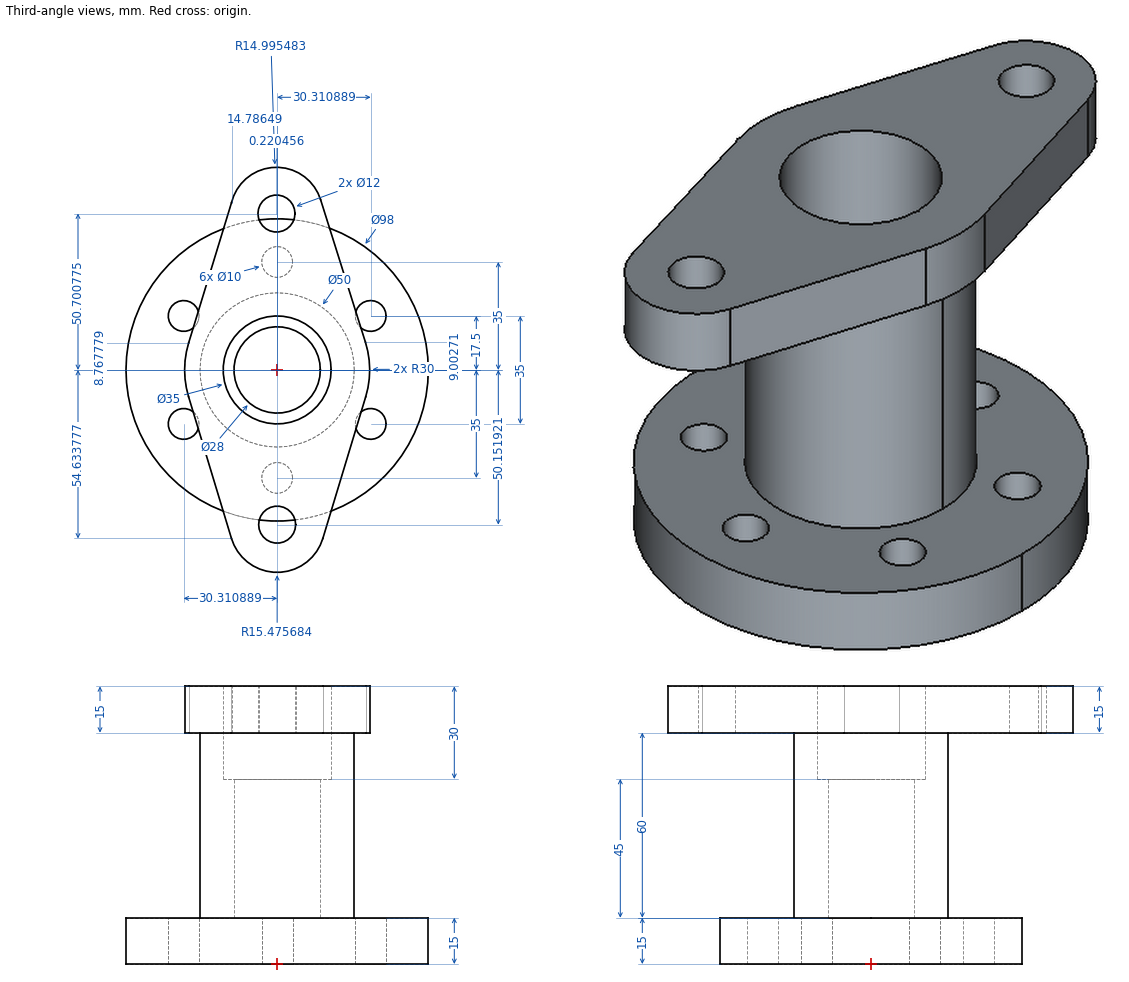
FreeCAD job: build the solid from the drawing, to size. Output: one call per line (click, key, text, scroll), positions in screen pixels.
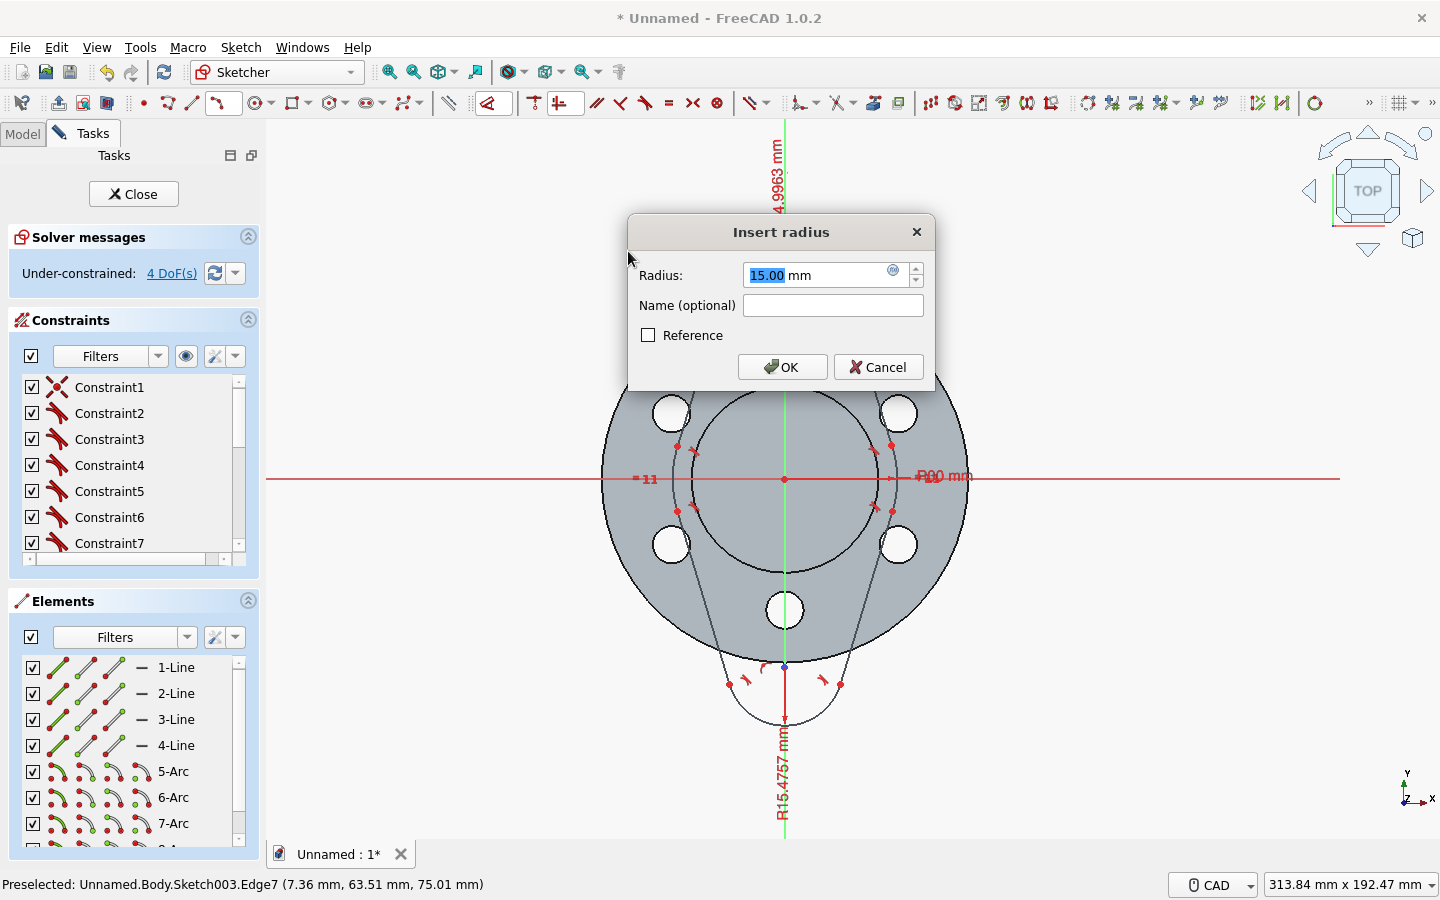
text(14.995483)
key(Return)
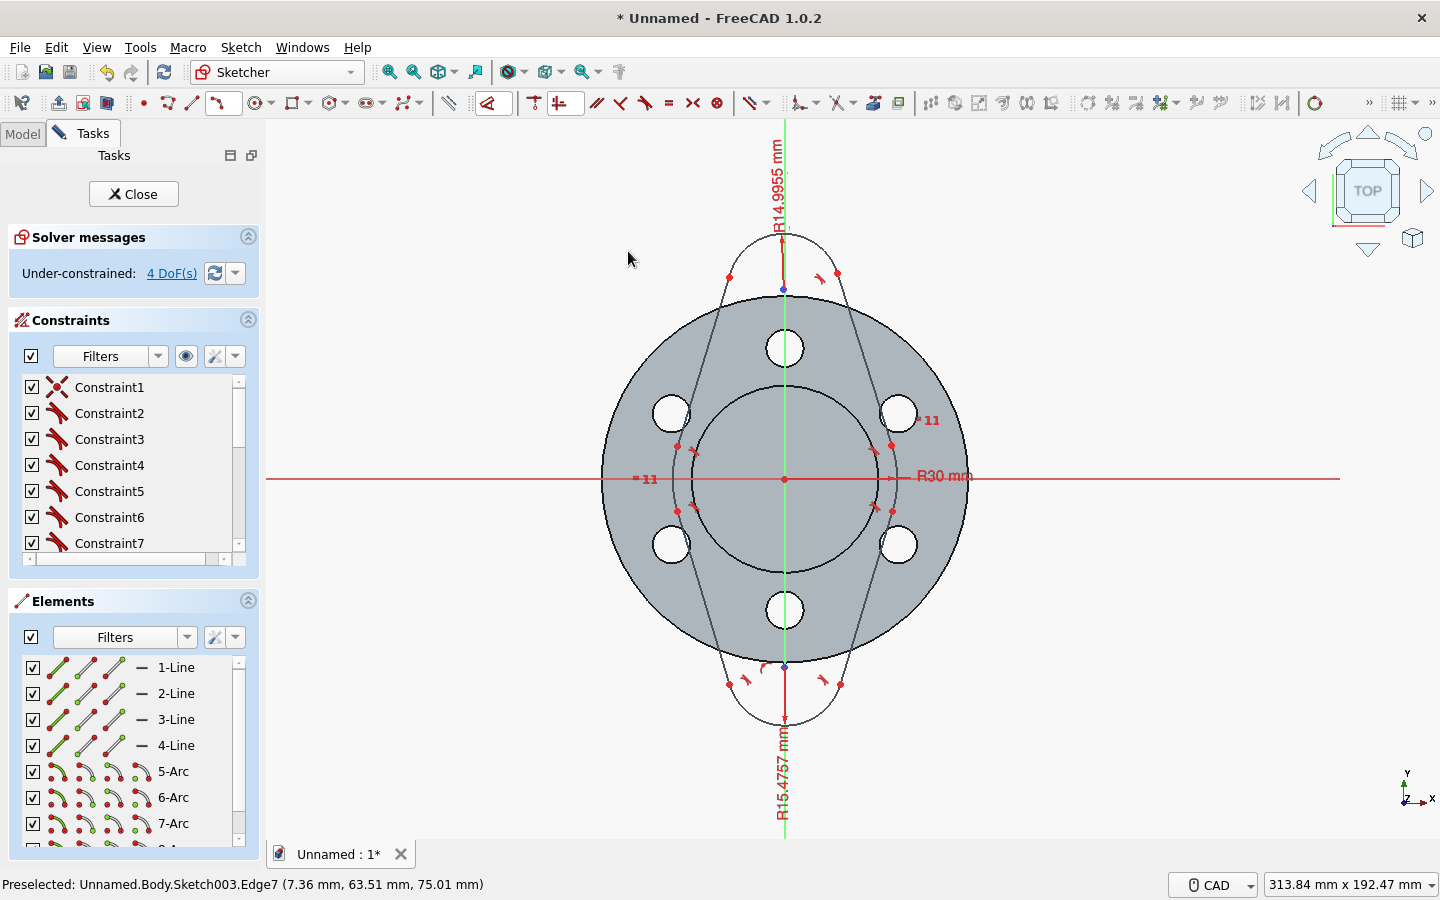
click(892, 445)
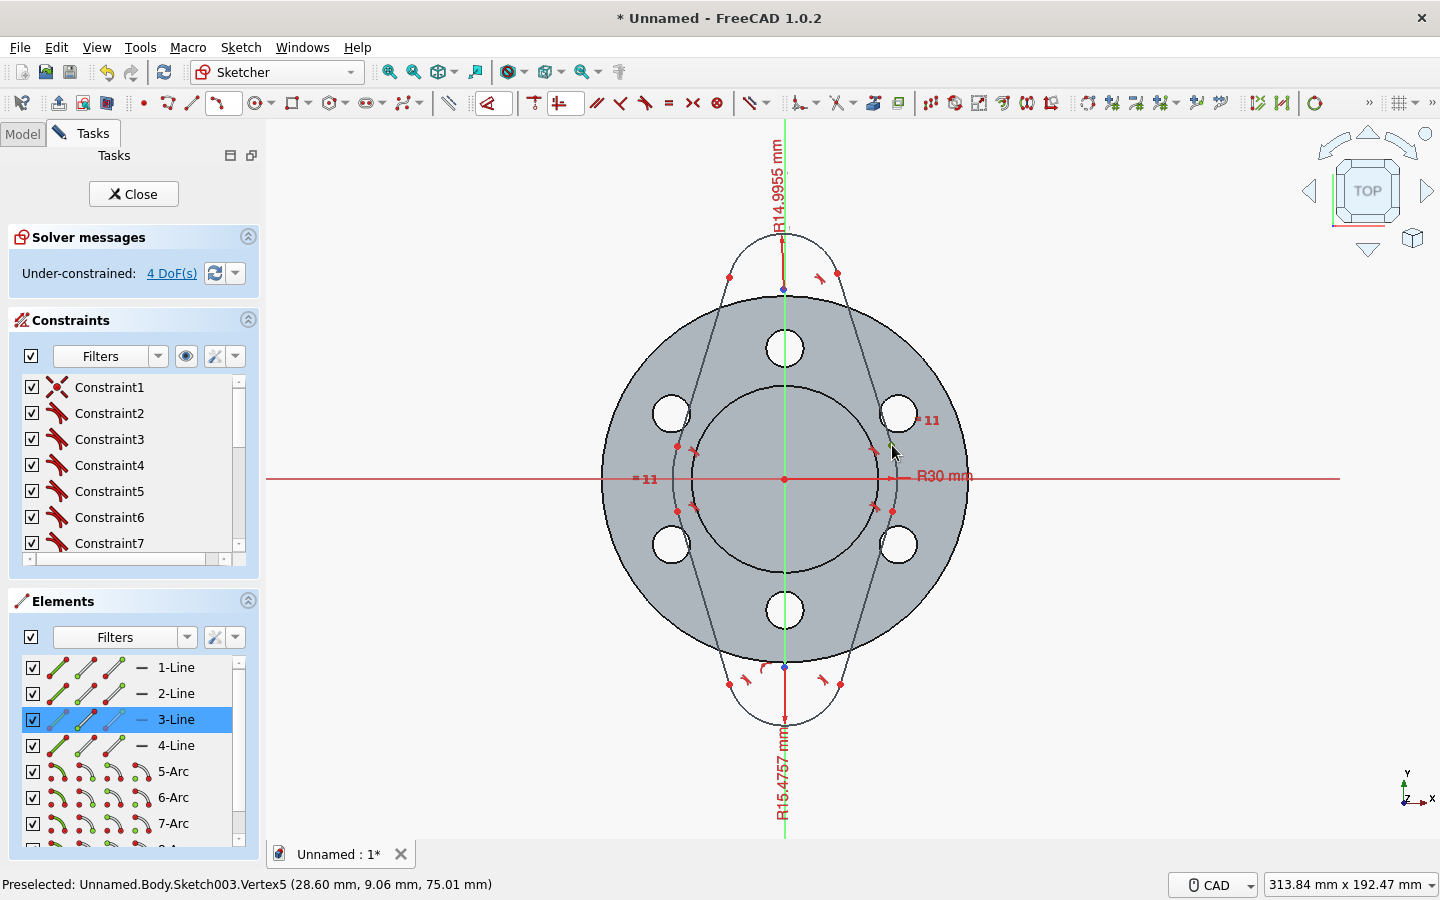
click(506, 104)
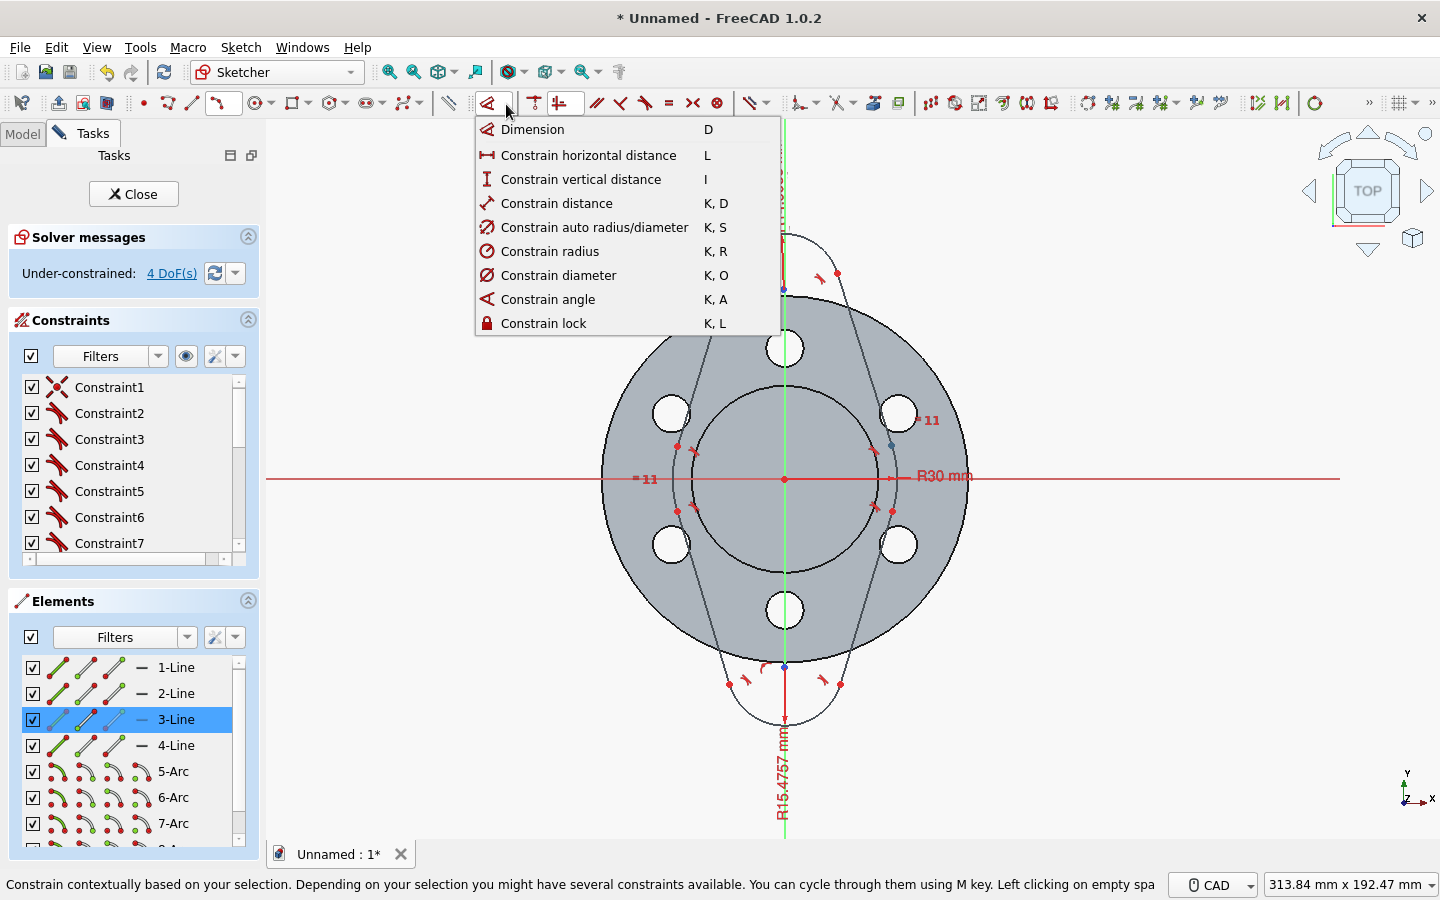
click(628, 179)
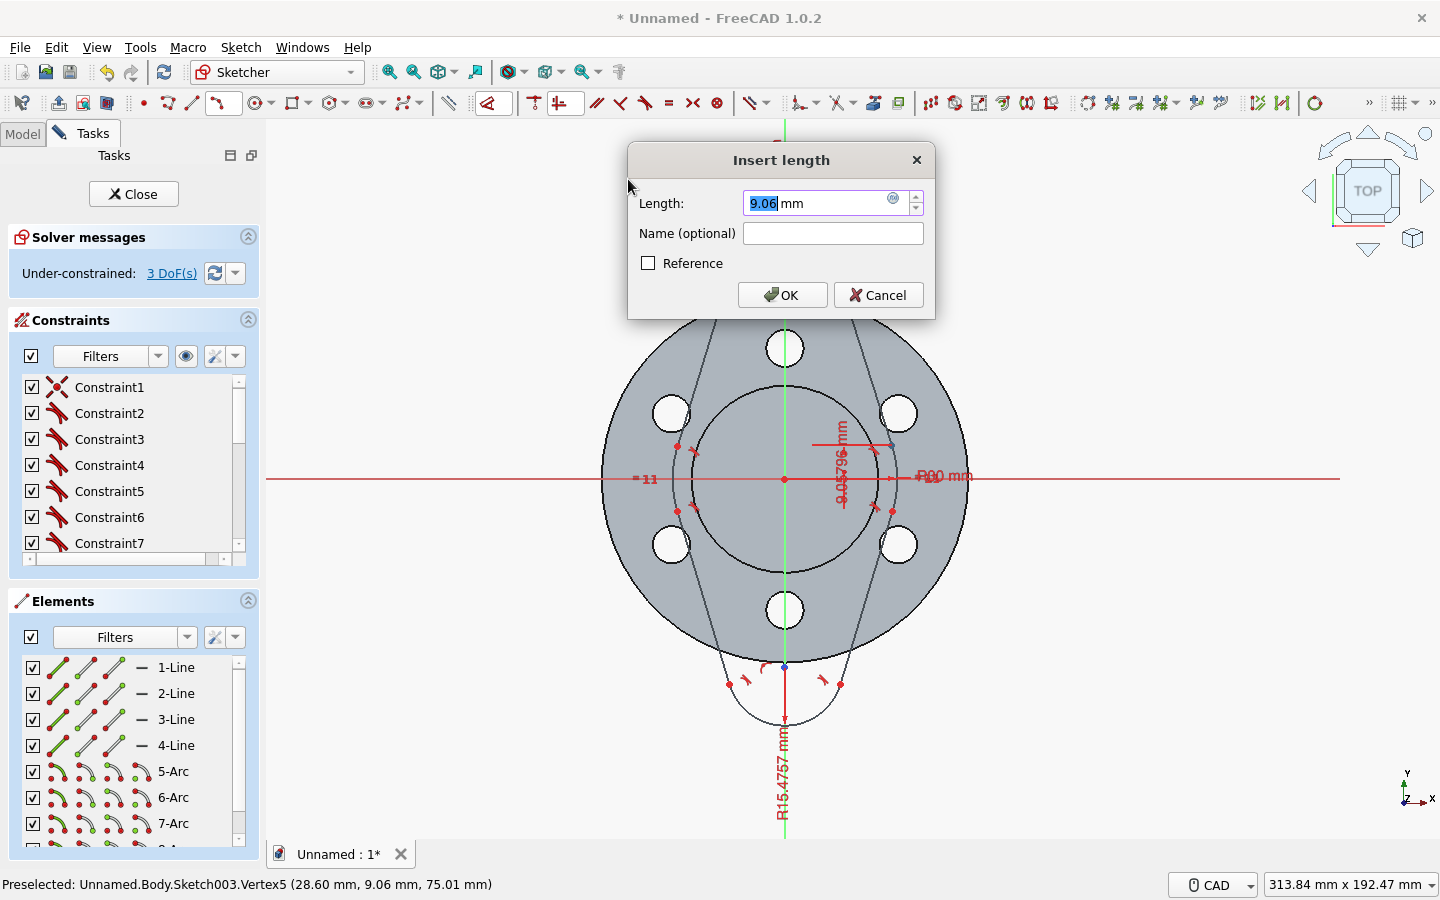
text(9.00271)
key(Return)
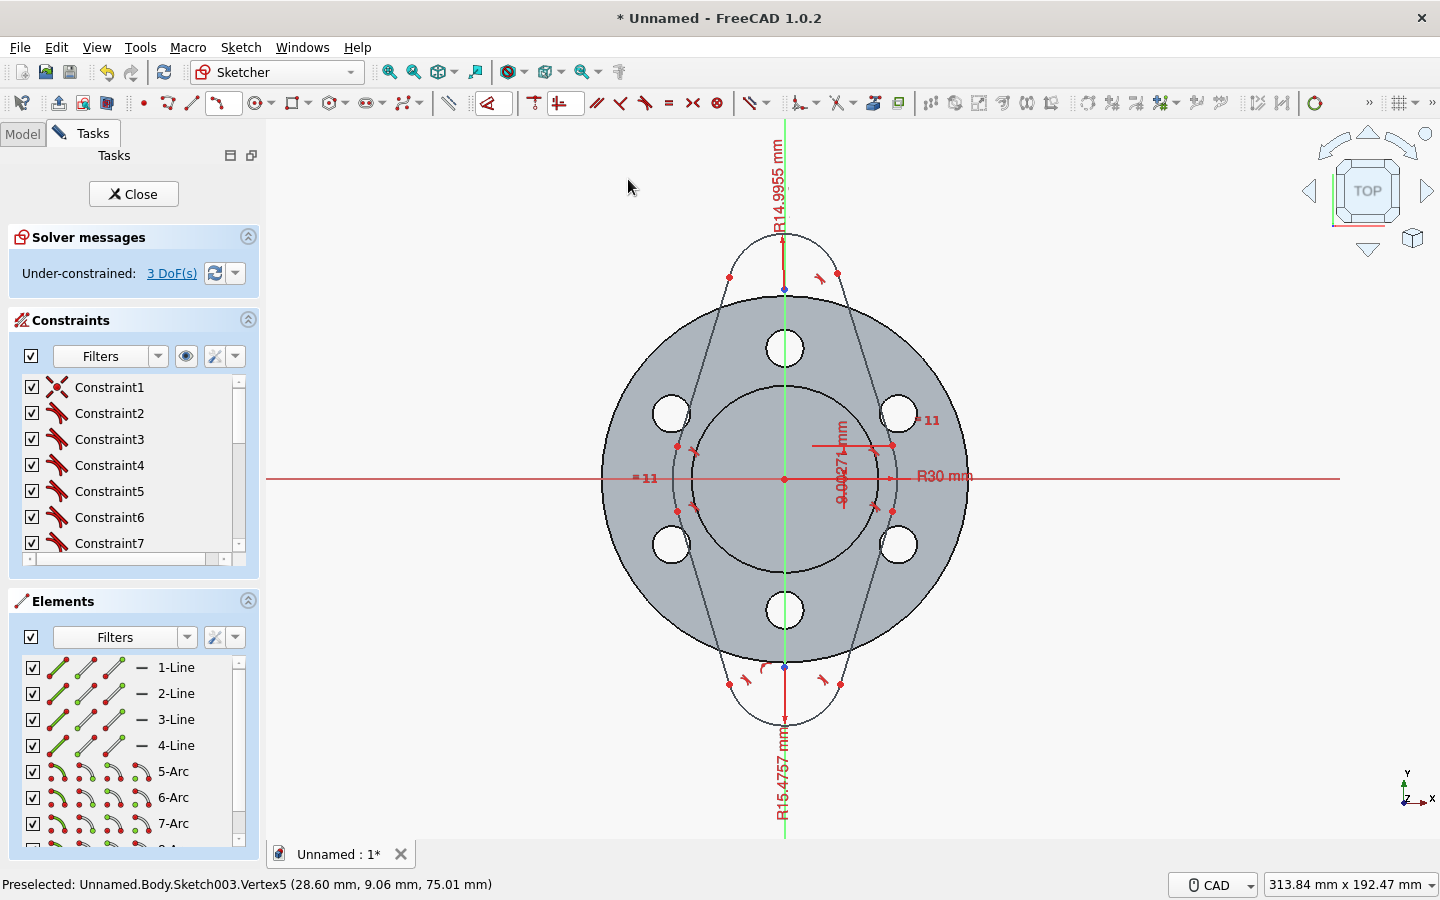
click(730, 277)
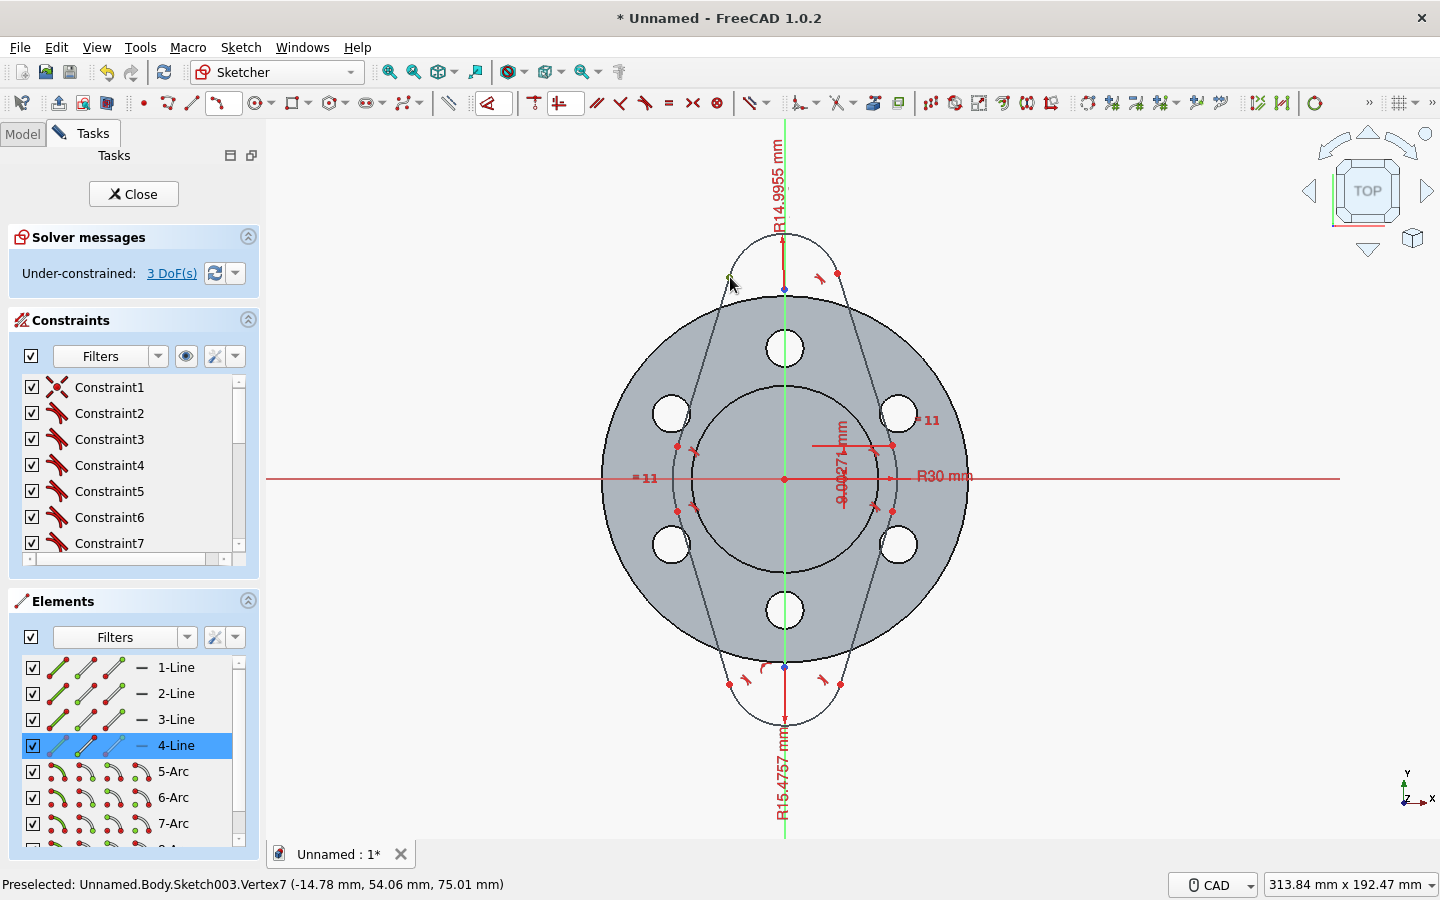
click(506, 104)